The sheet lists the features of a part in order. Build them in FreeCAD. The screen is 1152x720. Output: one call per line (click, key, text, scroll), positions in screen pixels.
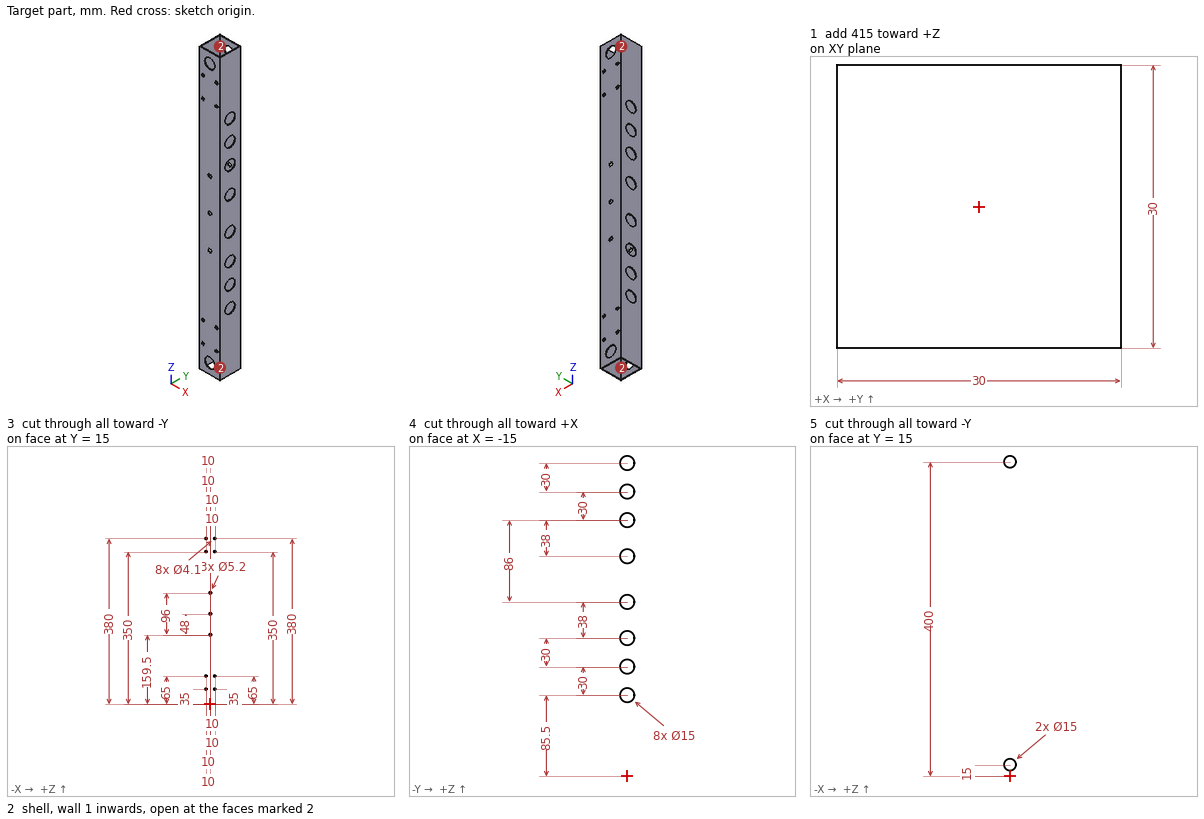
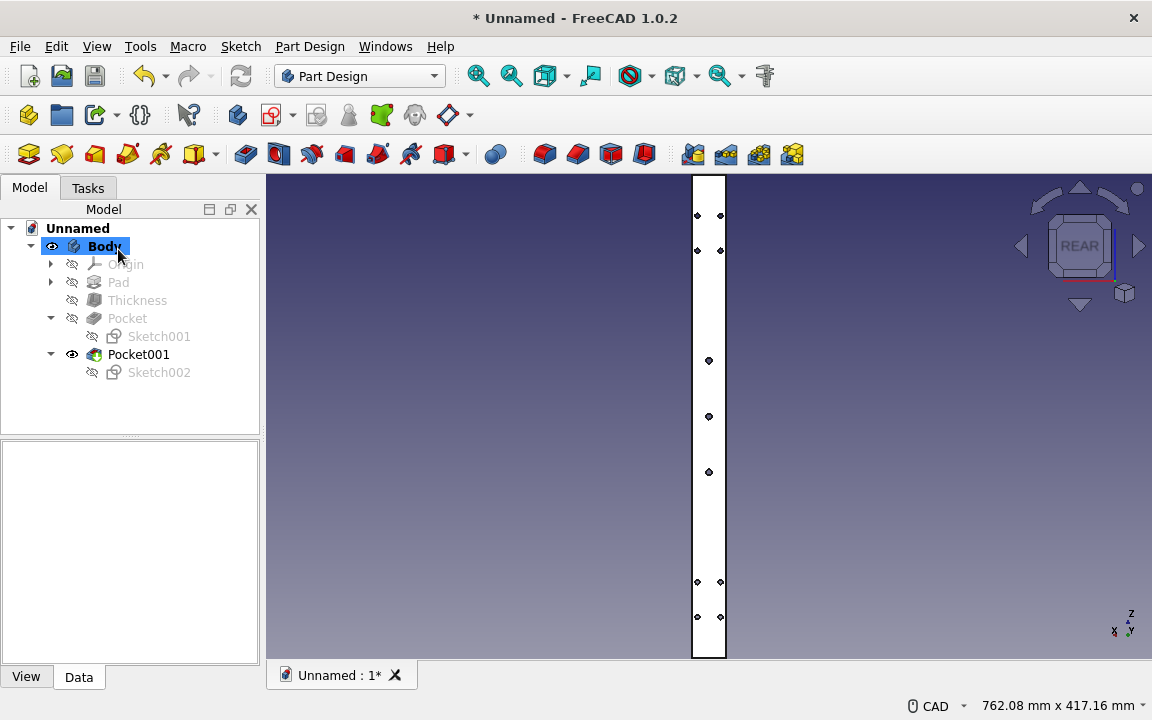
click(709, 278)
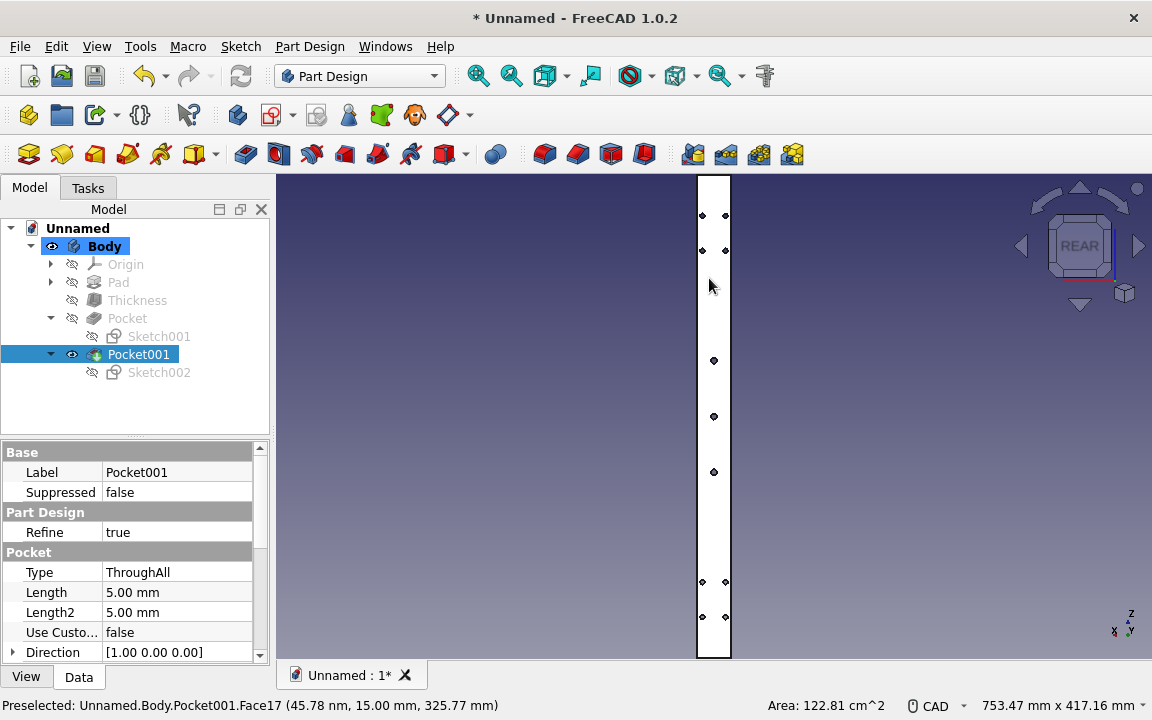
click(270, 116)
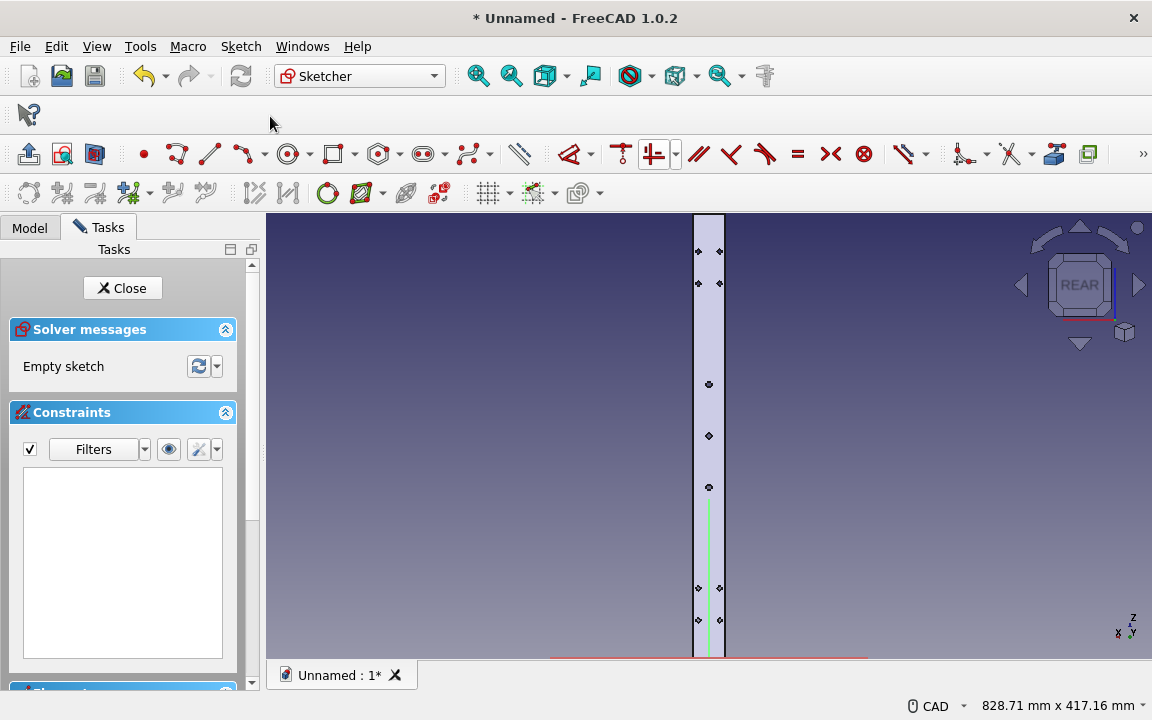
scroll(501, 428, down, 2)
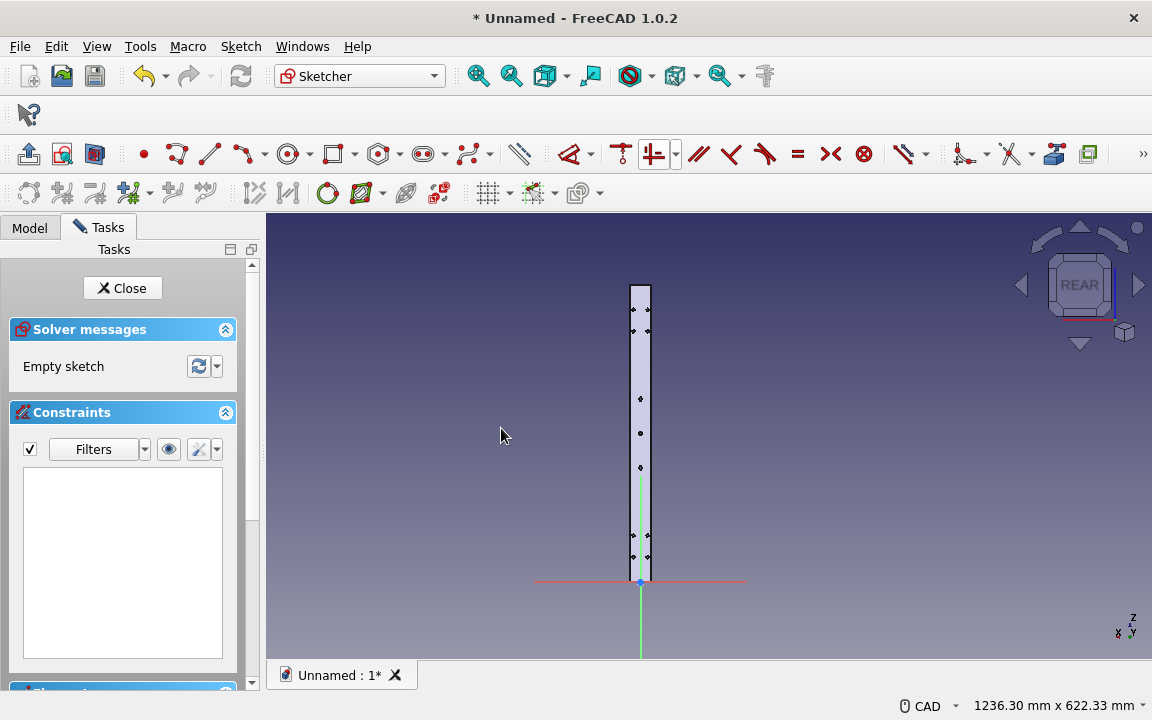
key(g)
key(c)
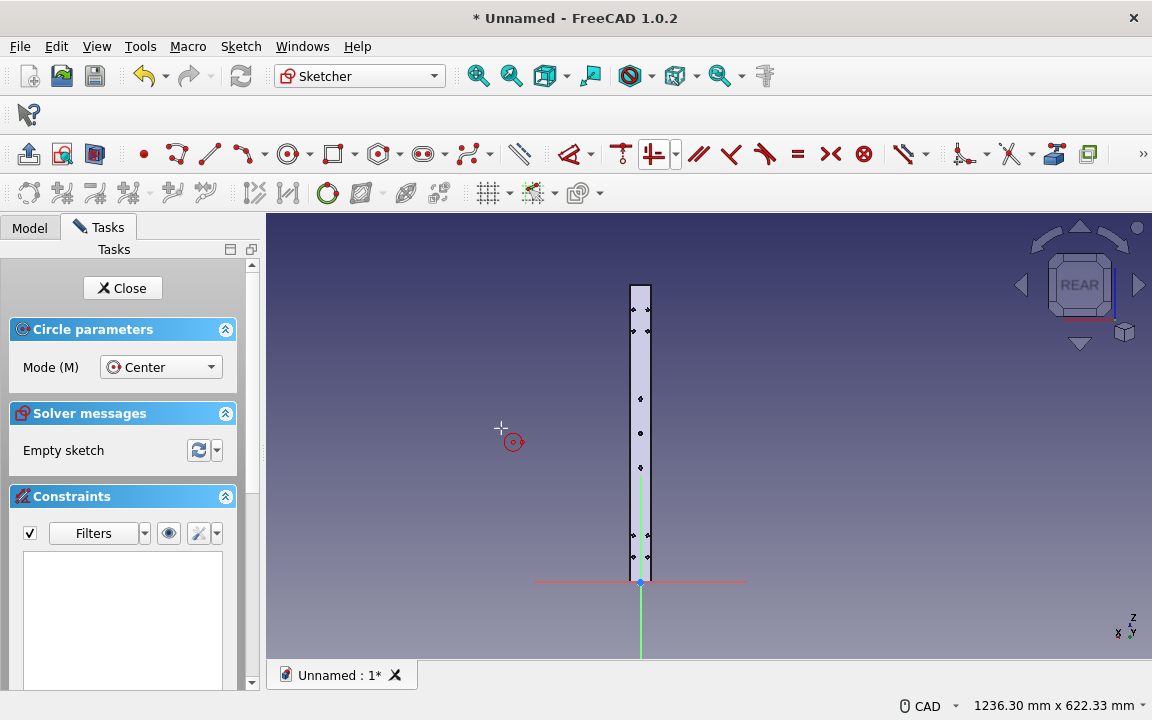
scroll(641, 571, up, 8)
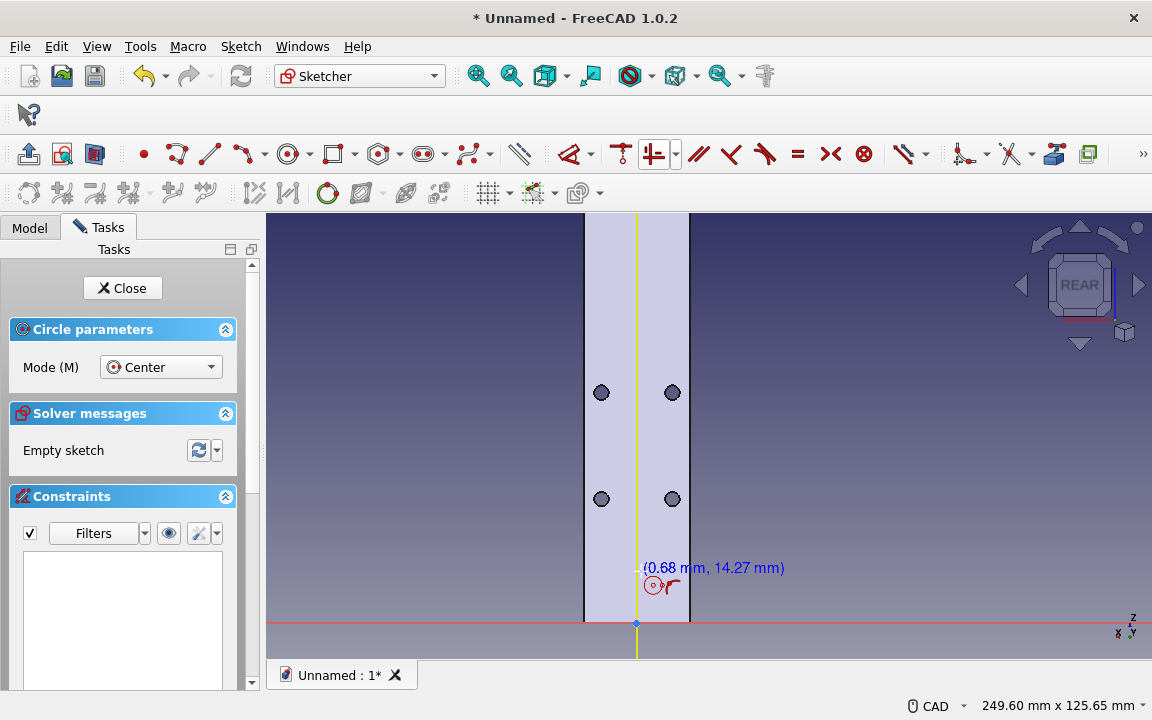
scroll(641, 572, down, 8)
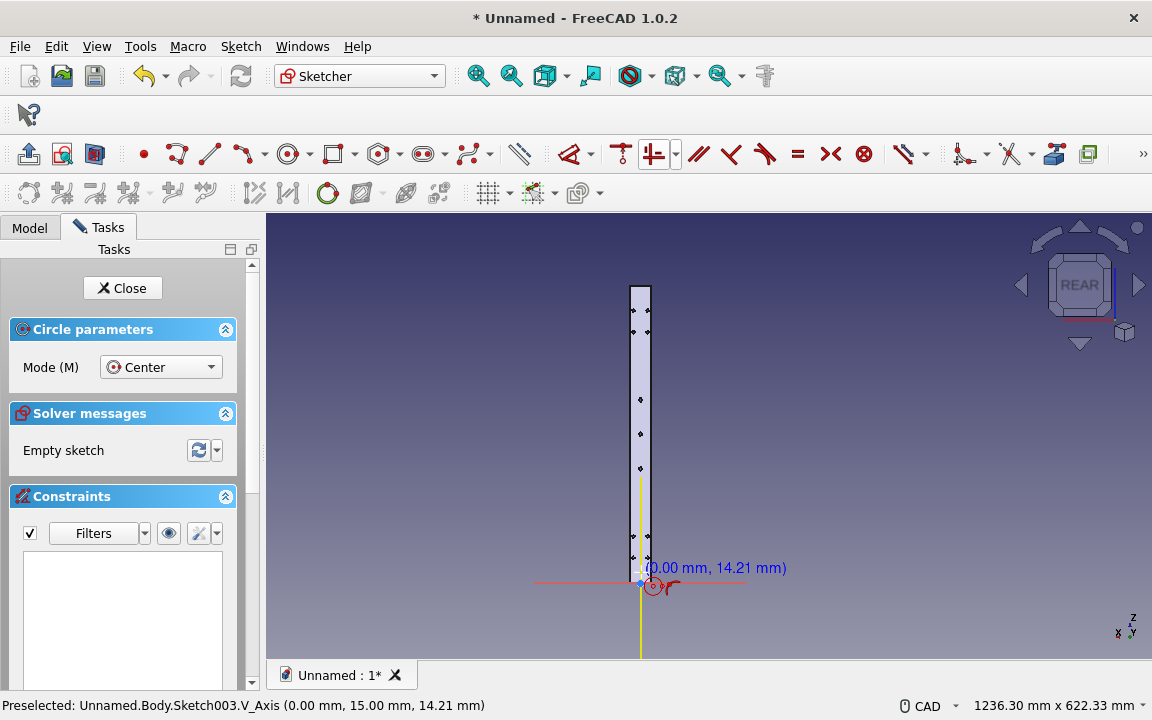
scroll(641, 572, up, 2)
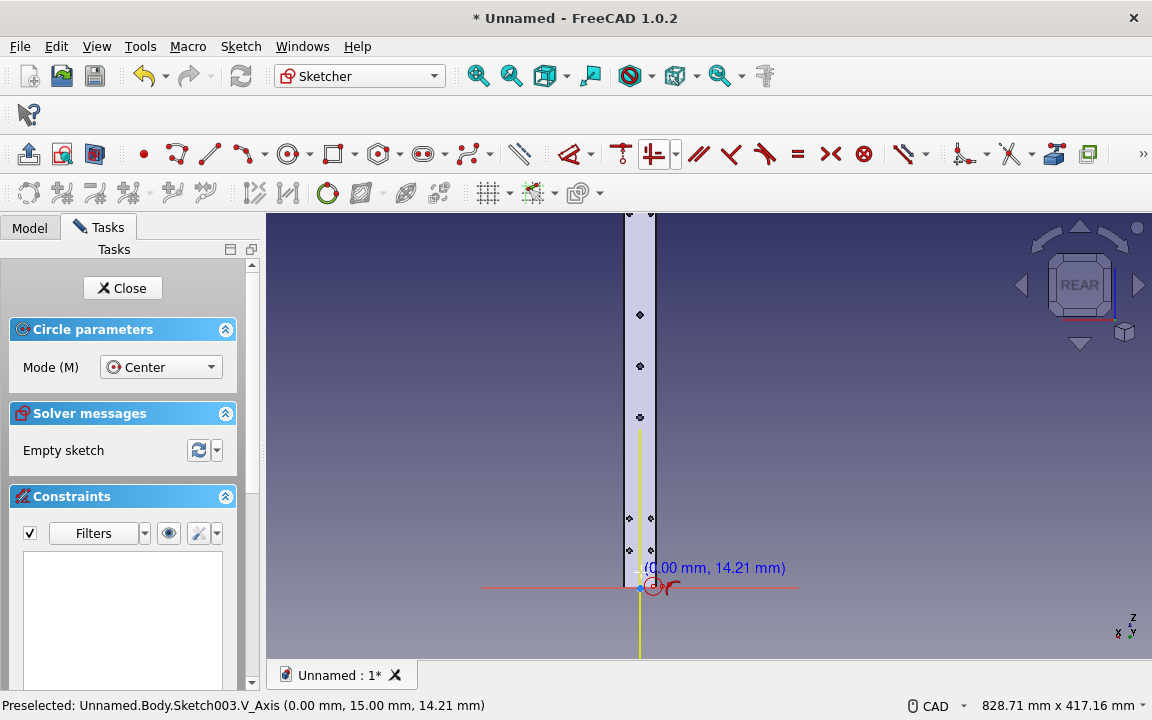
click(640, 572)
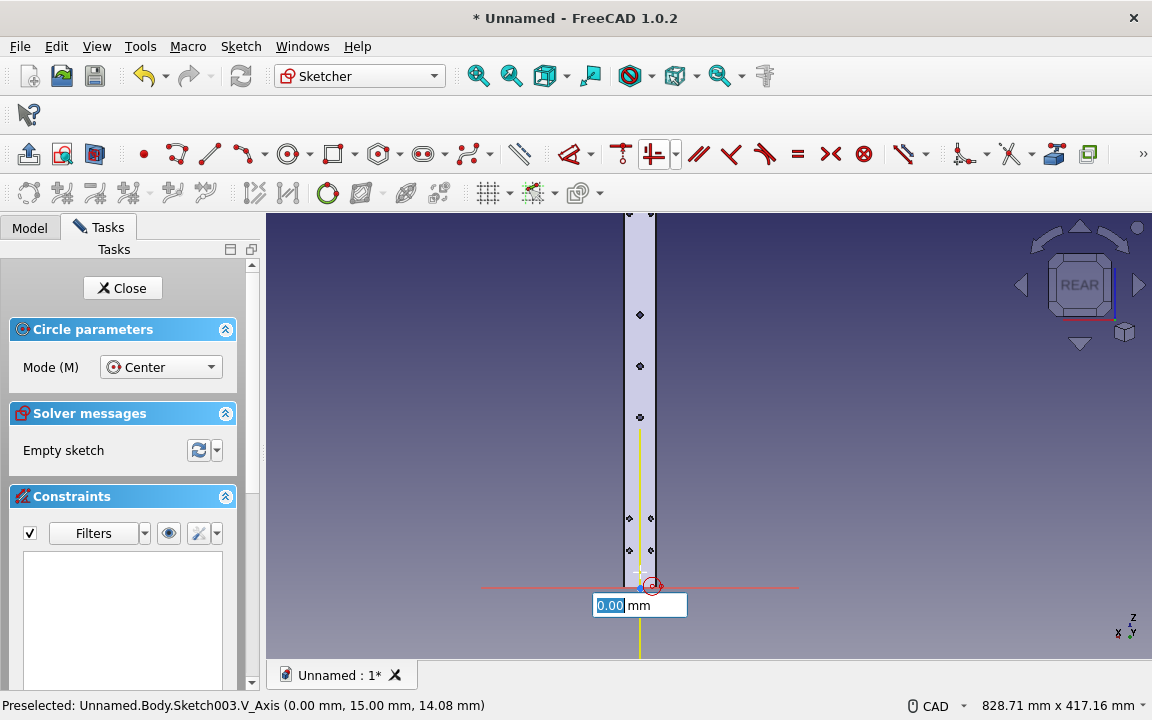
scroll(648, 569, up, 4)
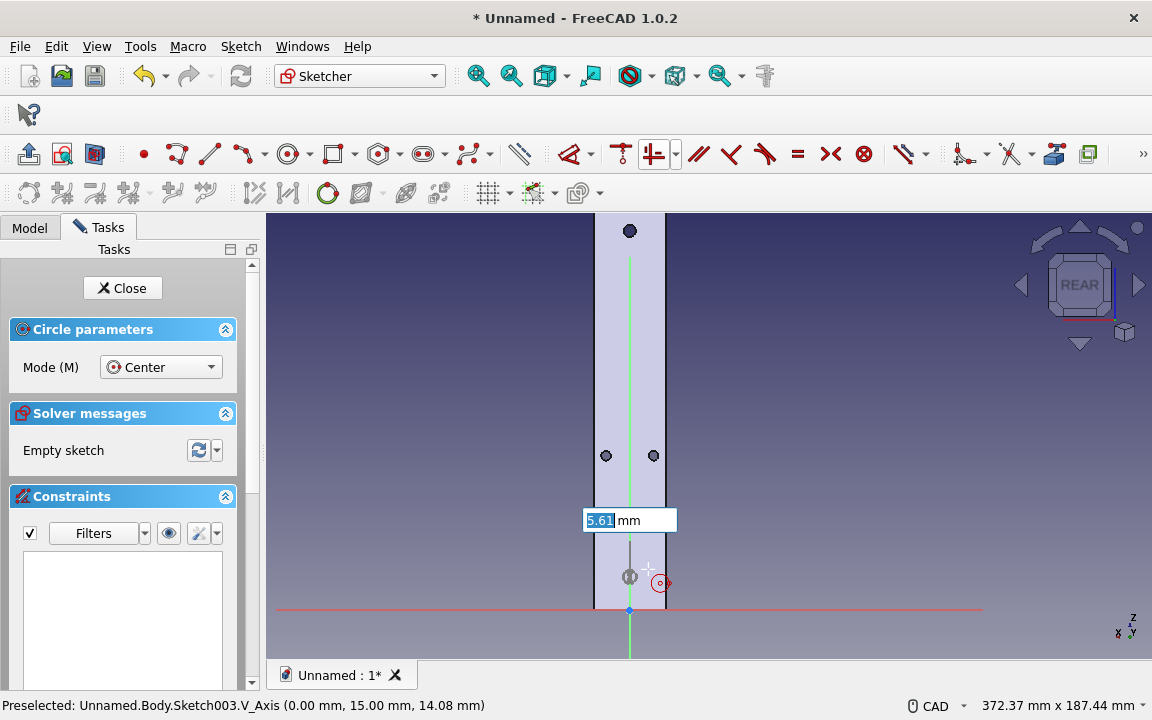
click(647, 569)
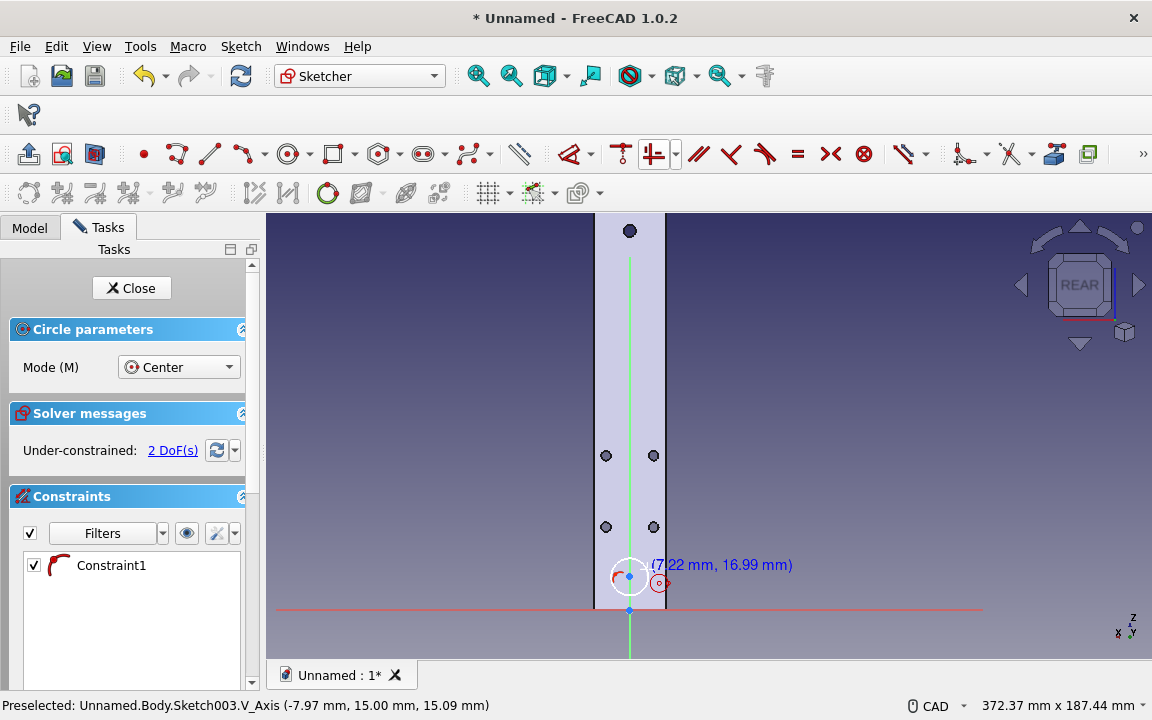
scroll(645, 570, down, 6)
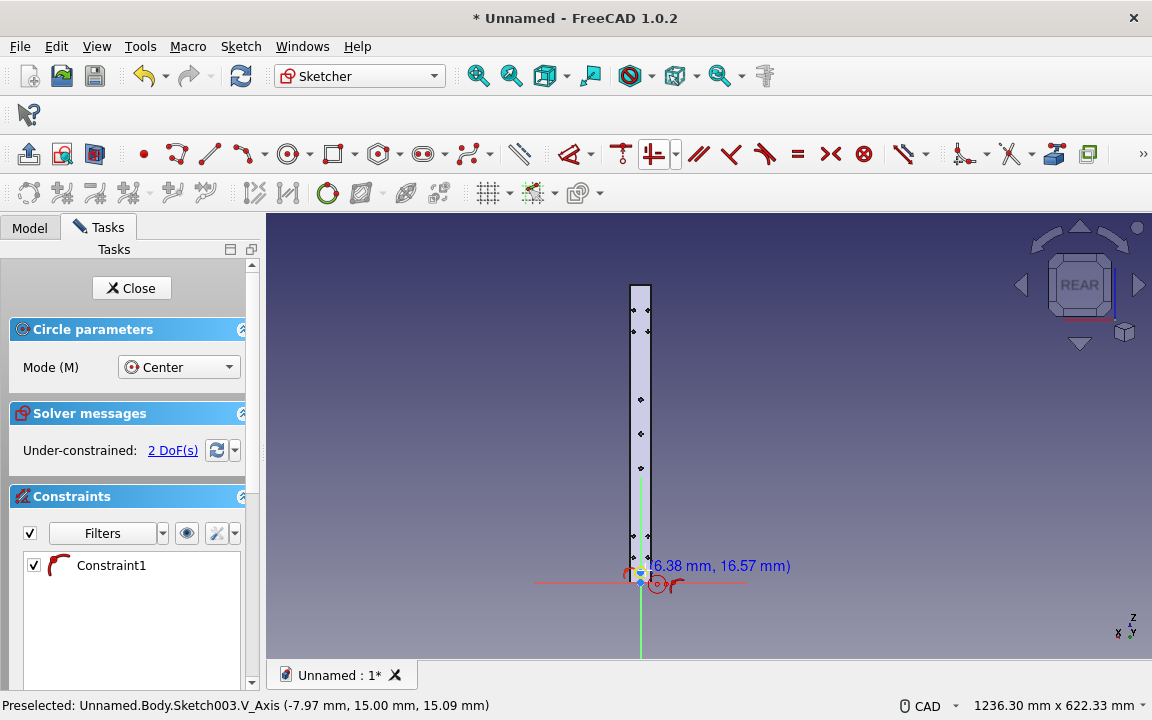
scroll(641, 296, up, 8)